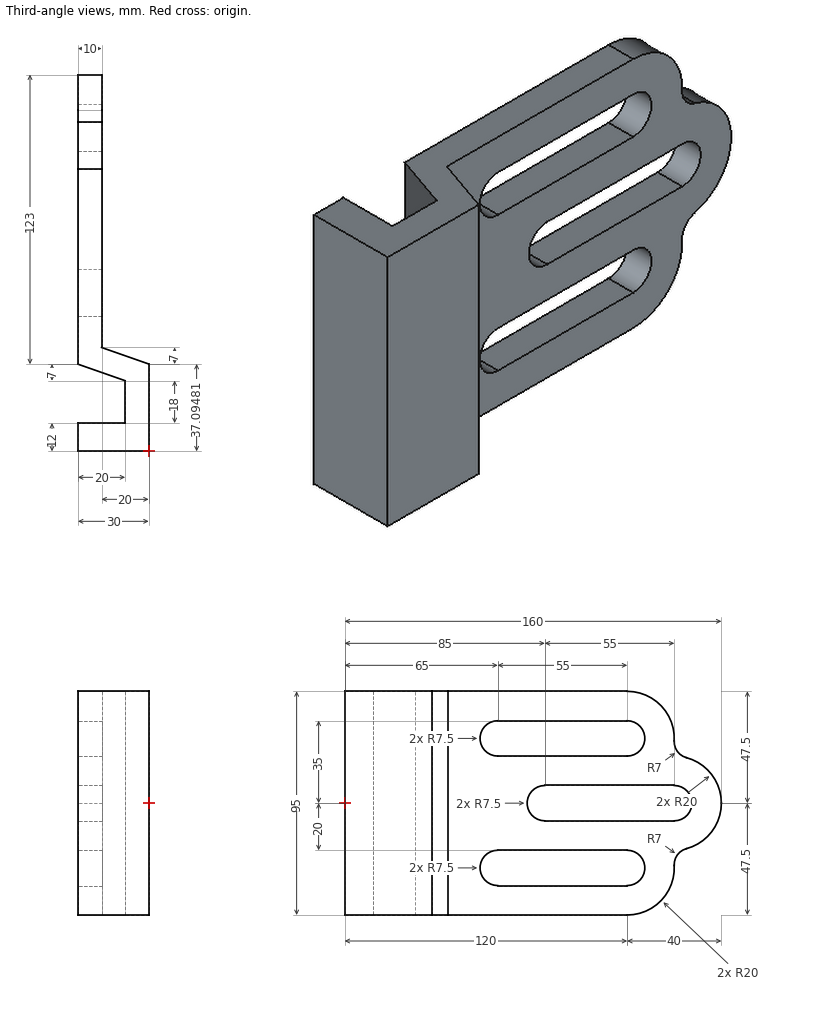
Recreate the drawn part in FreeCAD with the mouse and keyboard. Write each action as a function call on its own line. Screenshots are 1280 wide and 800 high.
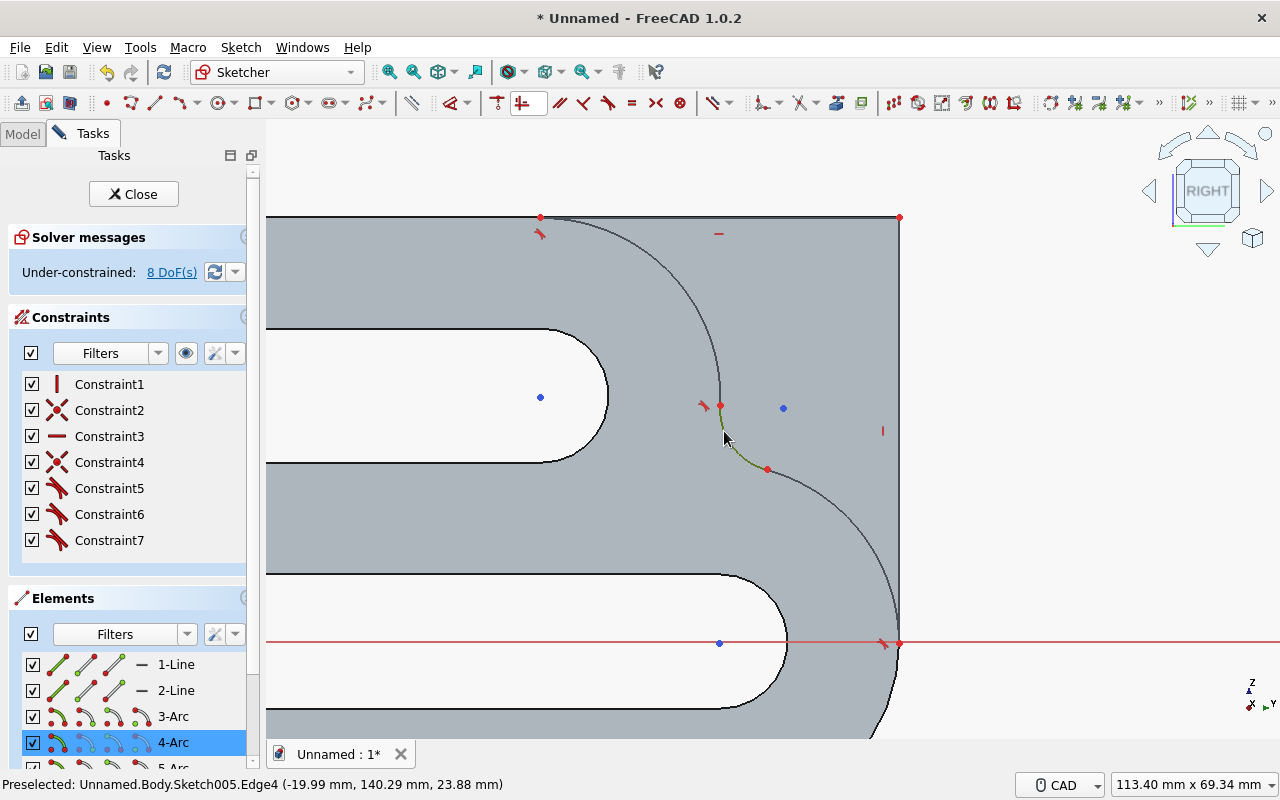
click(885, 575)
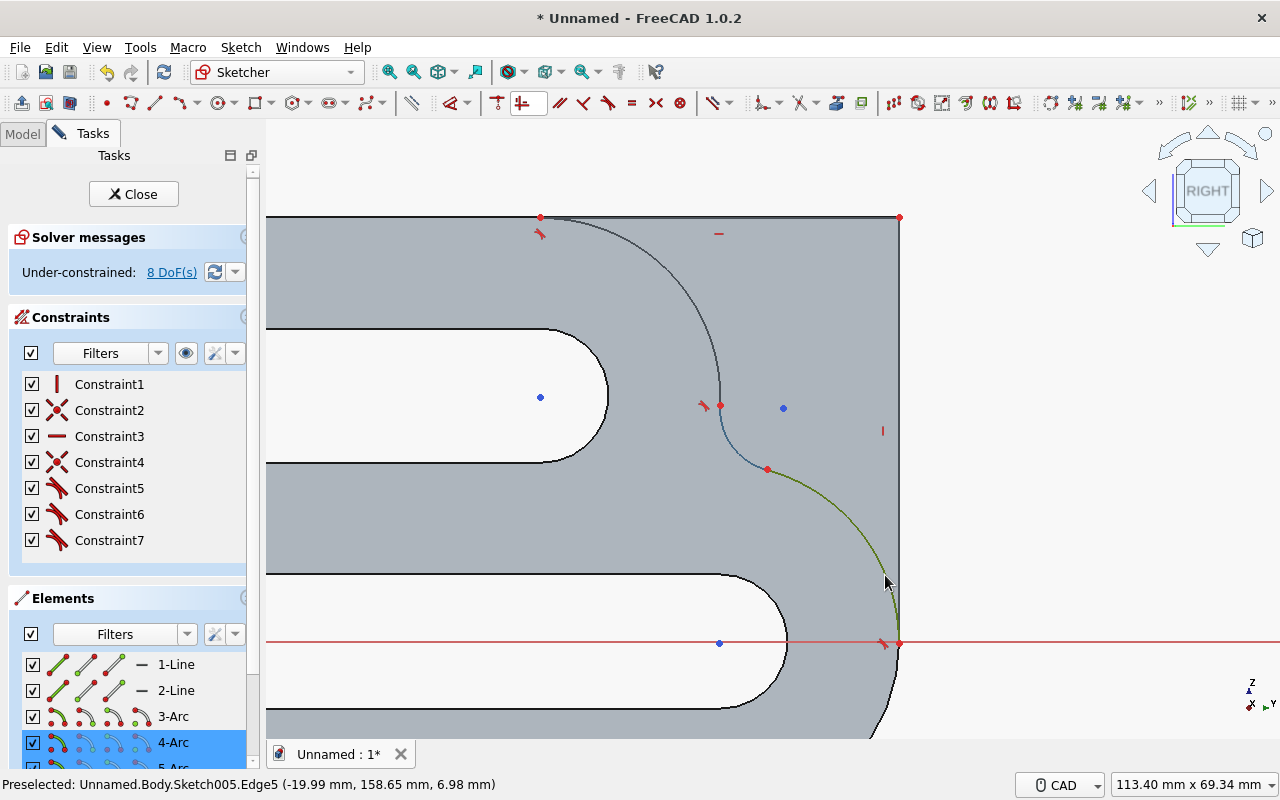
click(608, 104)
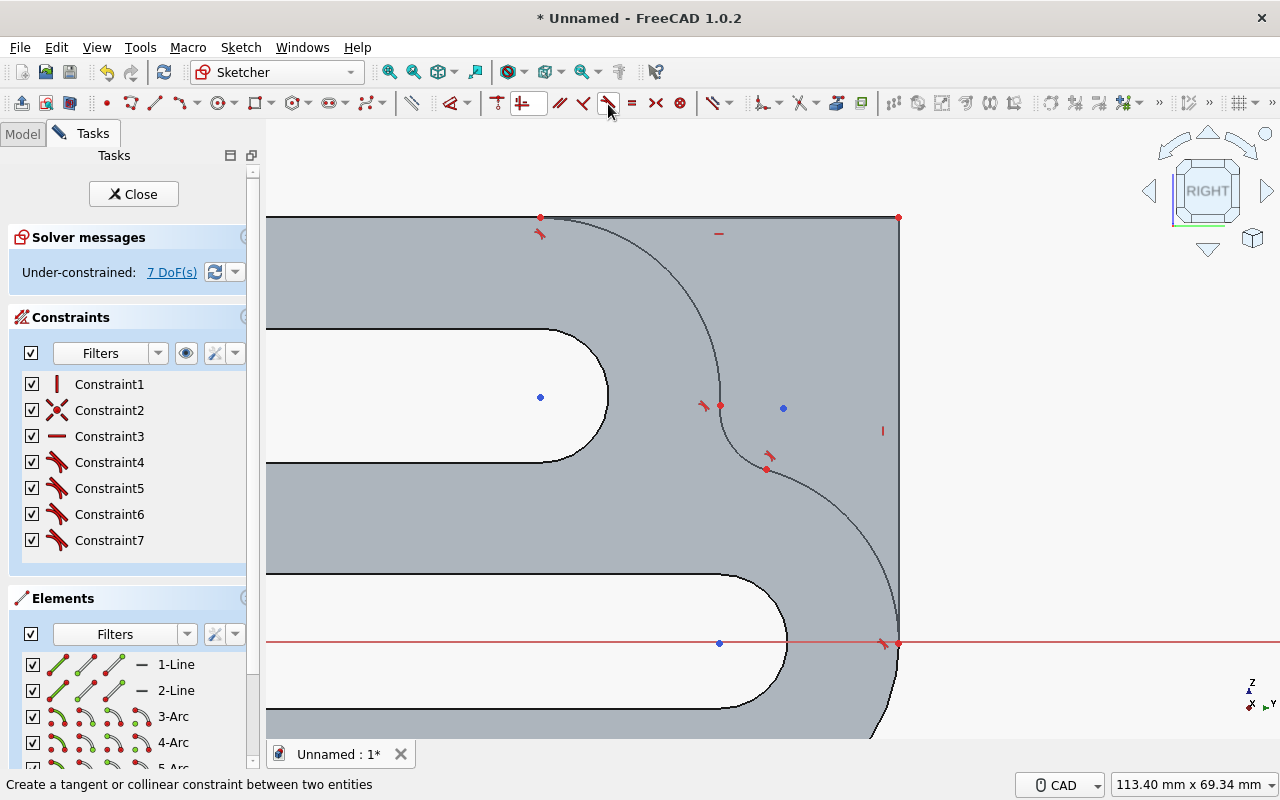
click(703, 321)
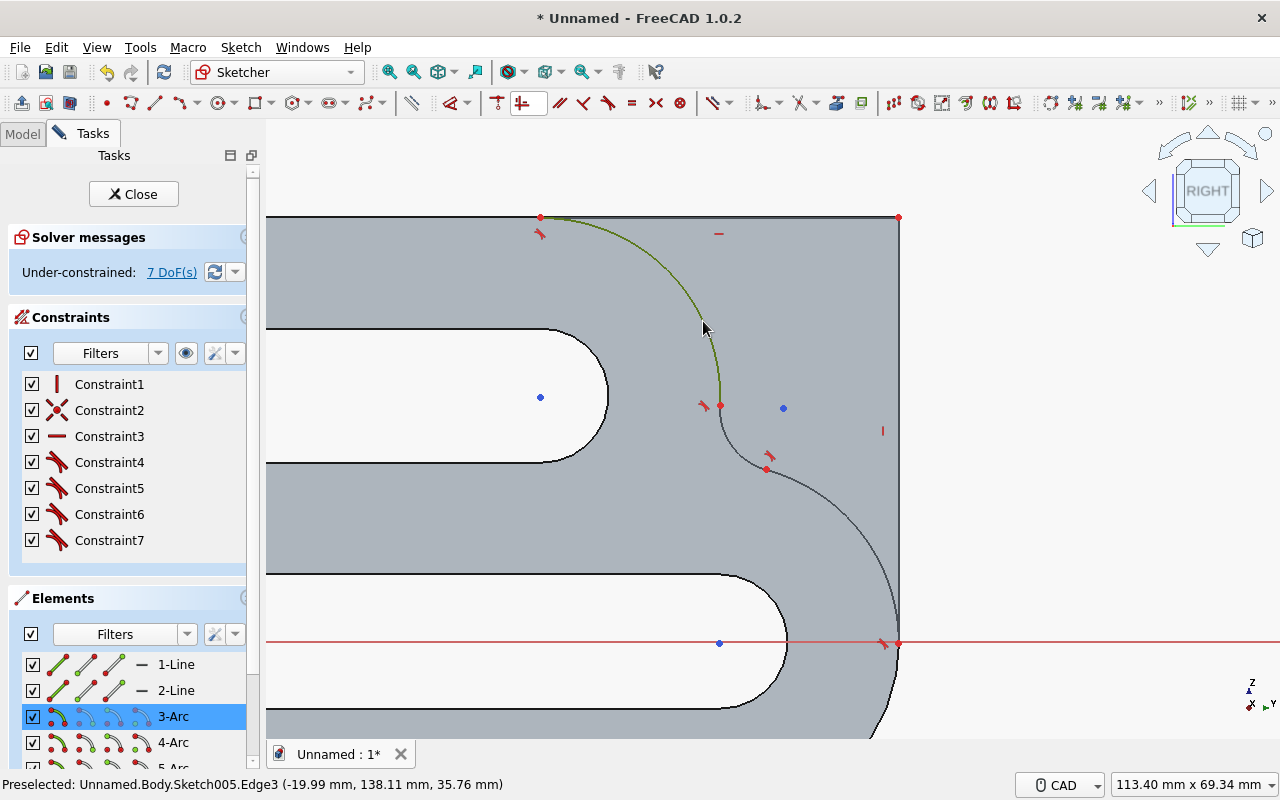
click(885, 575)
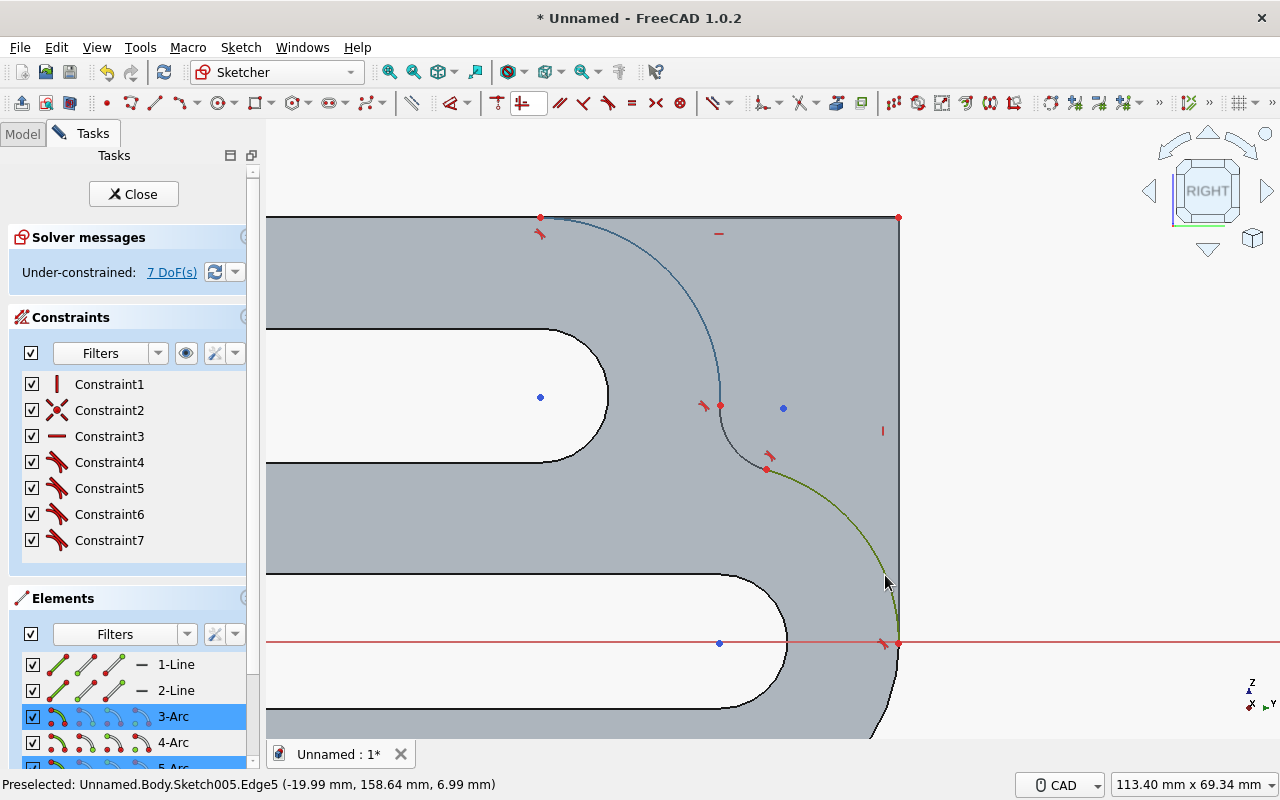
click(632, 104)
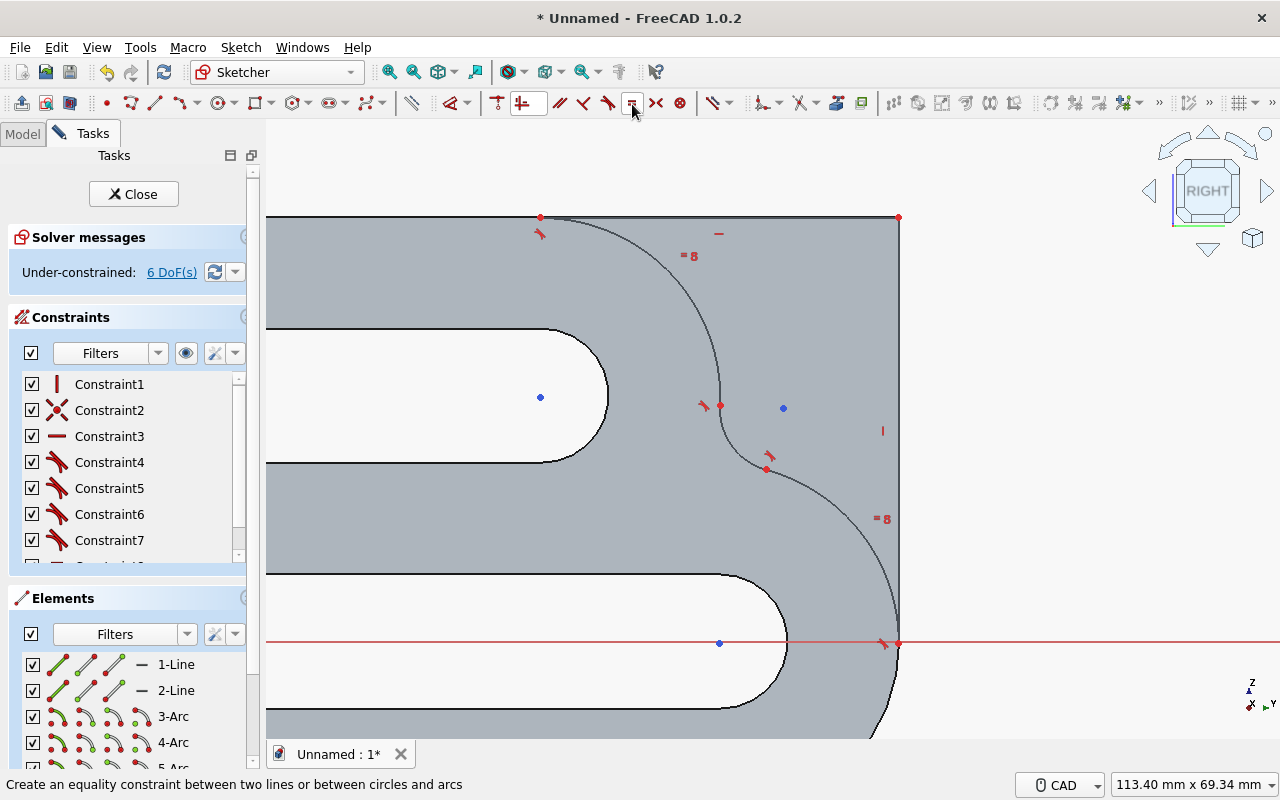
click(719, 643)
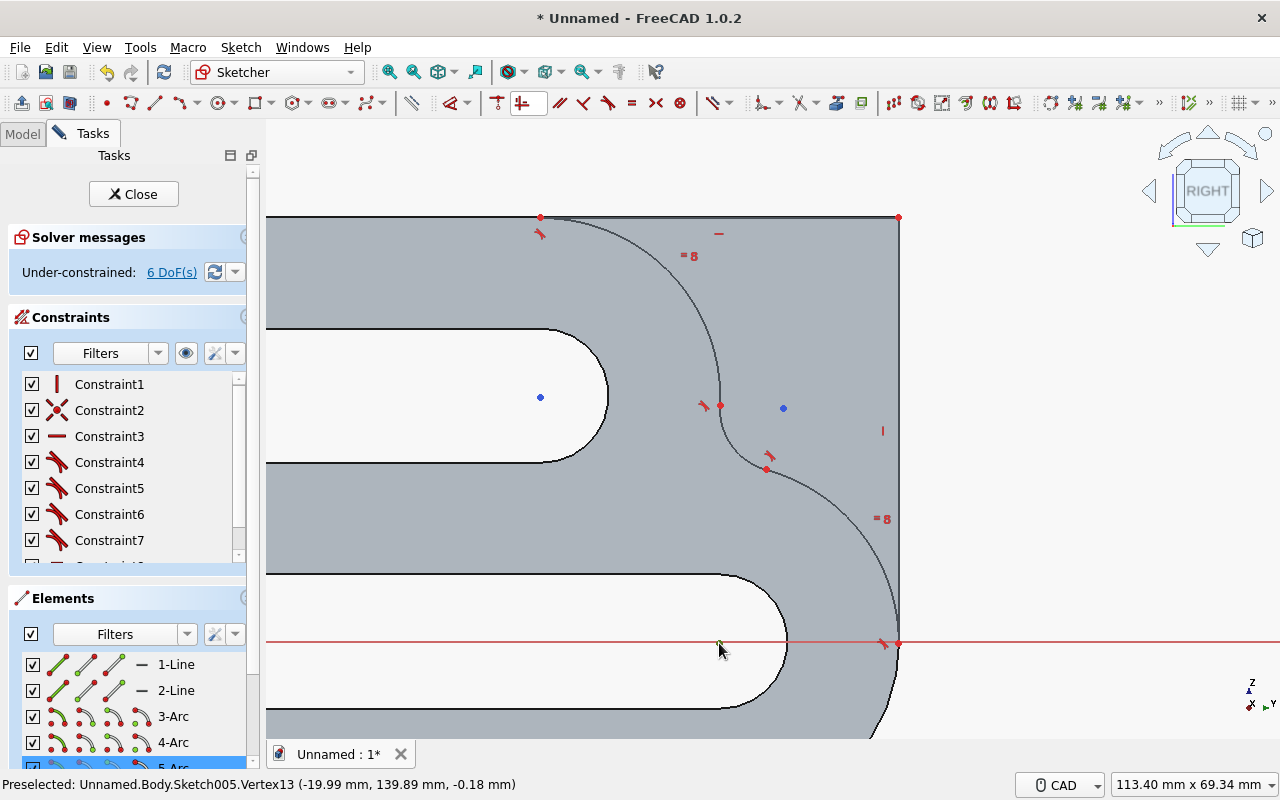
click(353, 642)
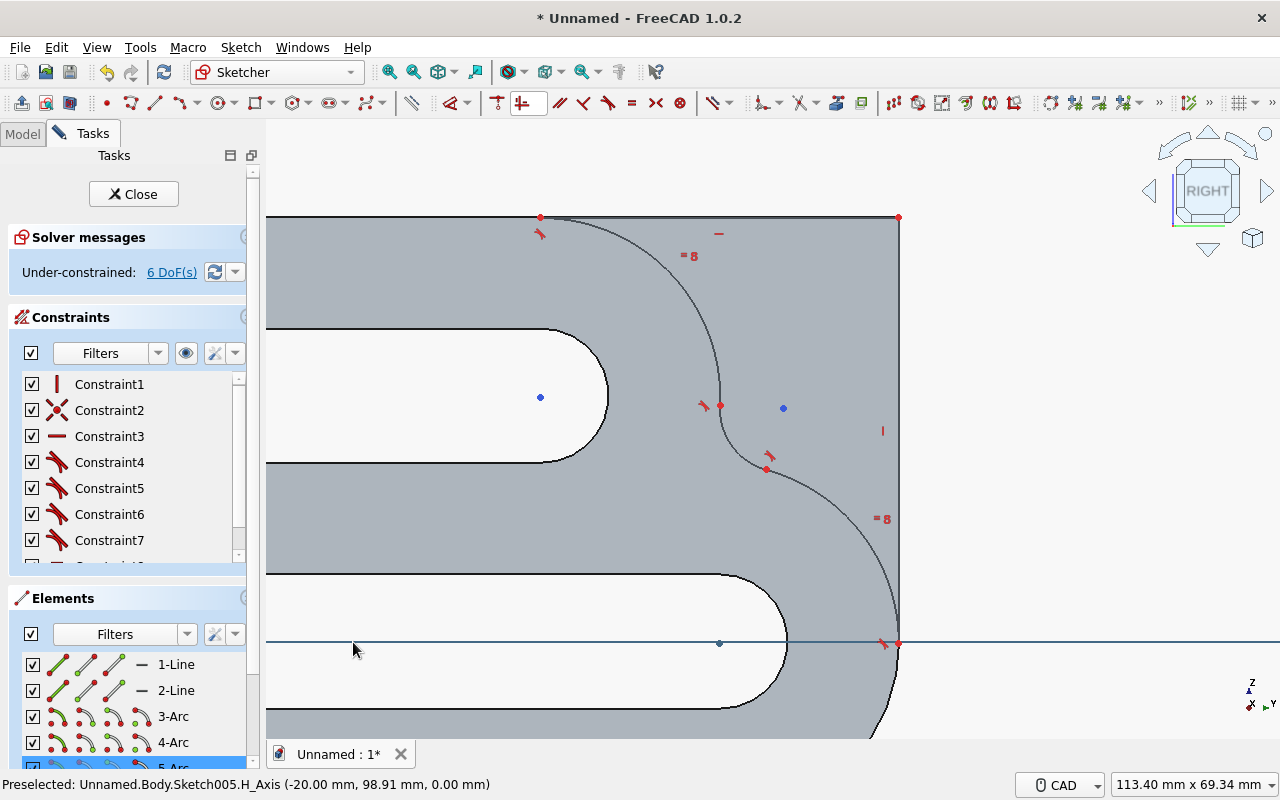
click(498, 104)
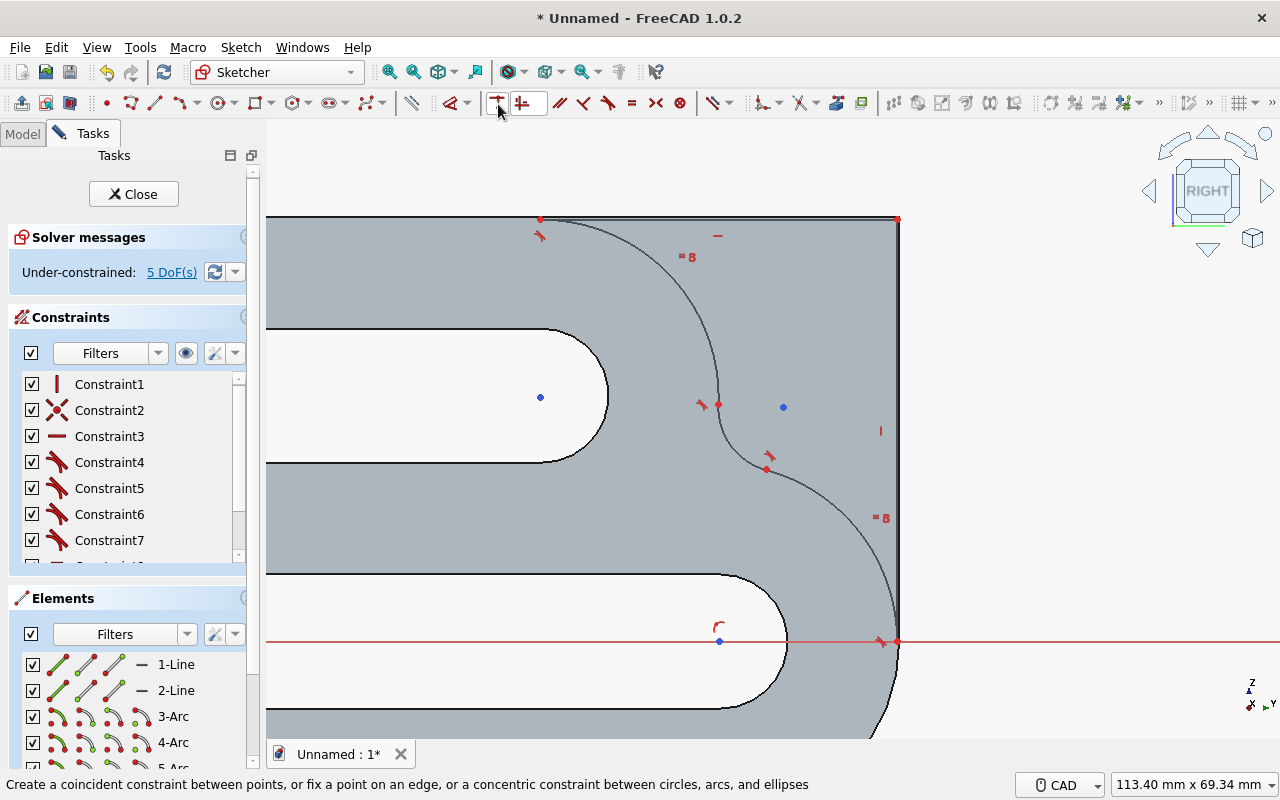
click(450, 104)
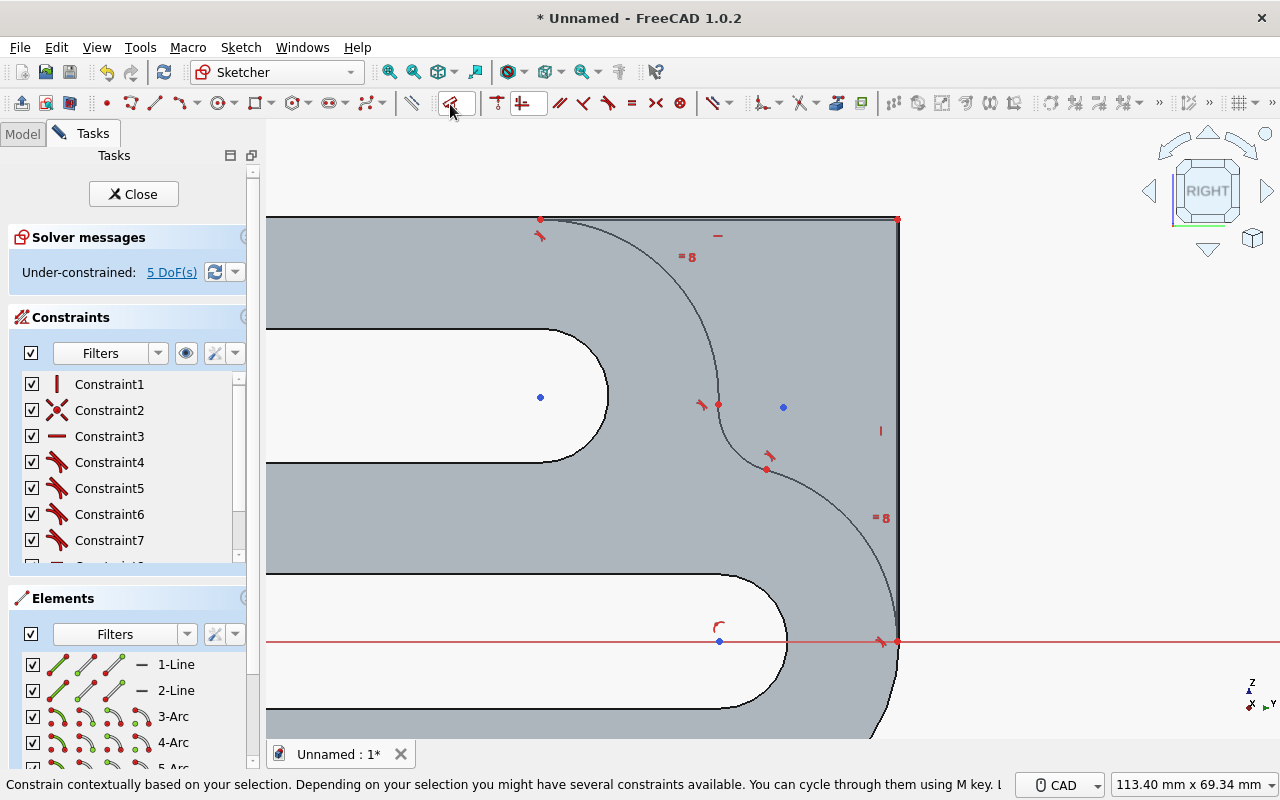
click(701, 321)
click(730, 307)